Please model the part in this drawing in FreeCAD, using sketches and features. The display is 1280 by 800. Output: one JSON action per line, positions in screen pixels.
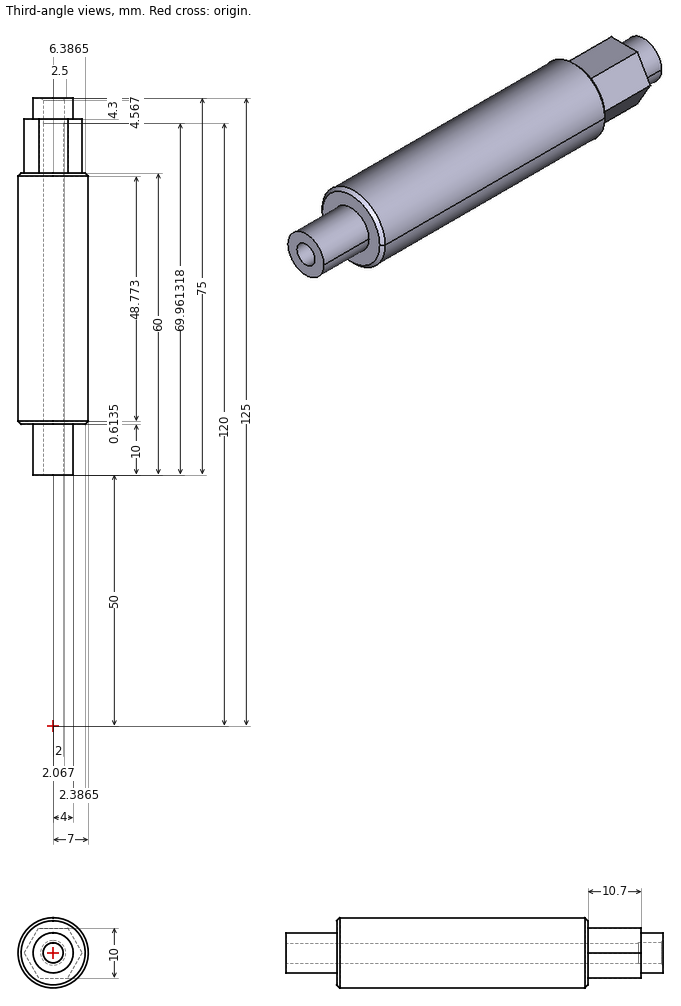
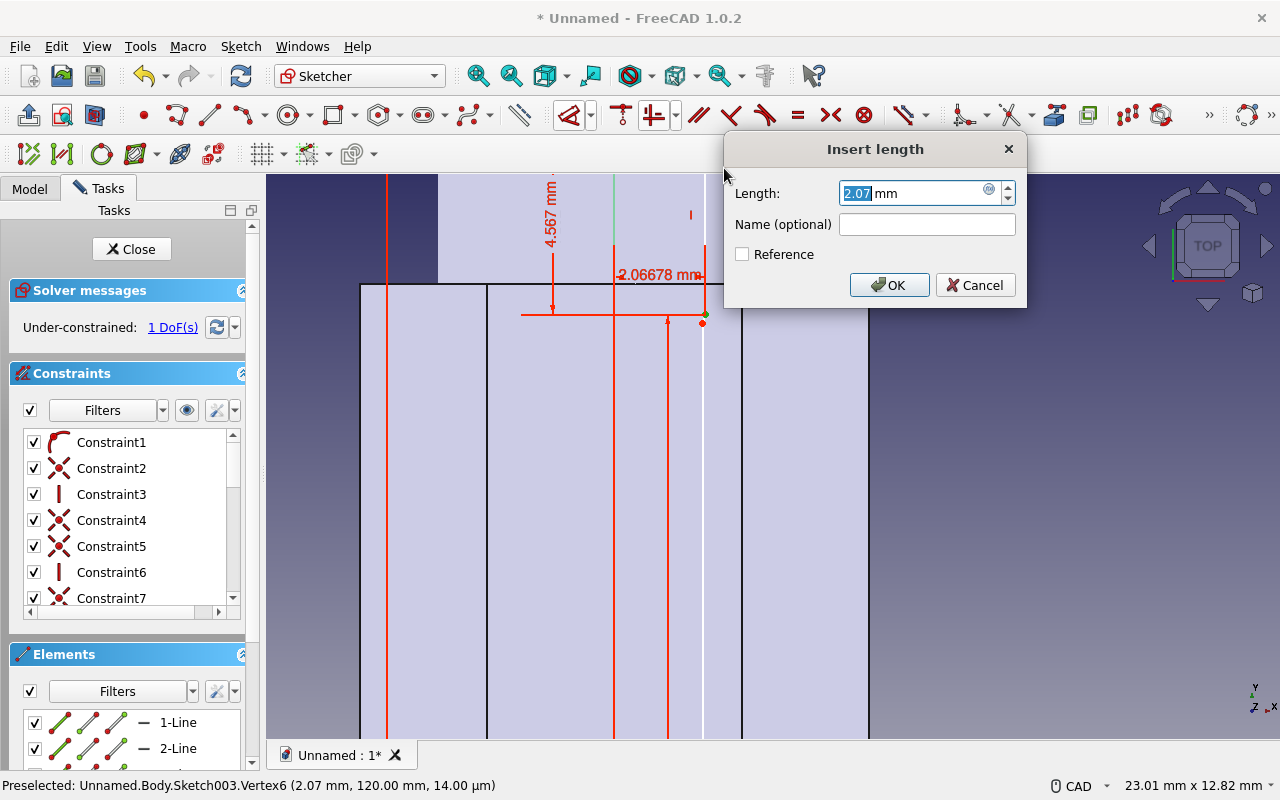
{"action": "type", "text": "2.067"}
{"action": "key", "text": "Return"}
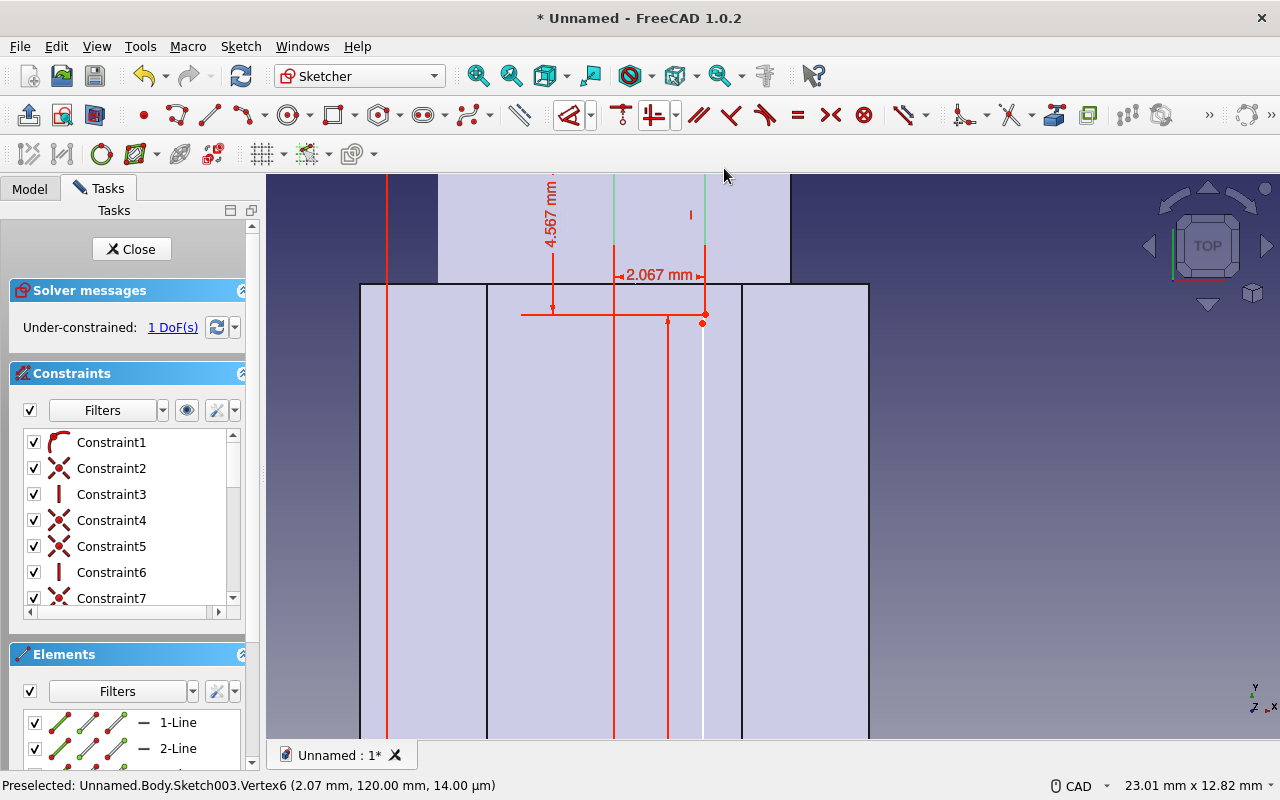
{"action": "scroll", "coordinate": [707, 302], "scroll_direction": "down", "scroll_amount": 14}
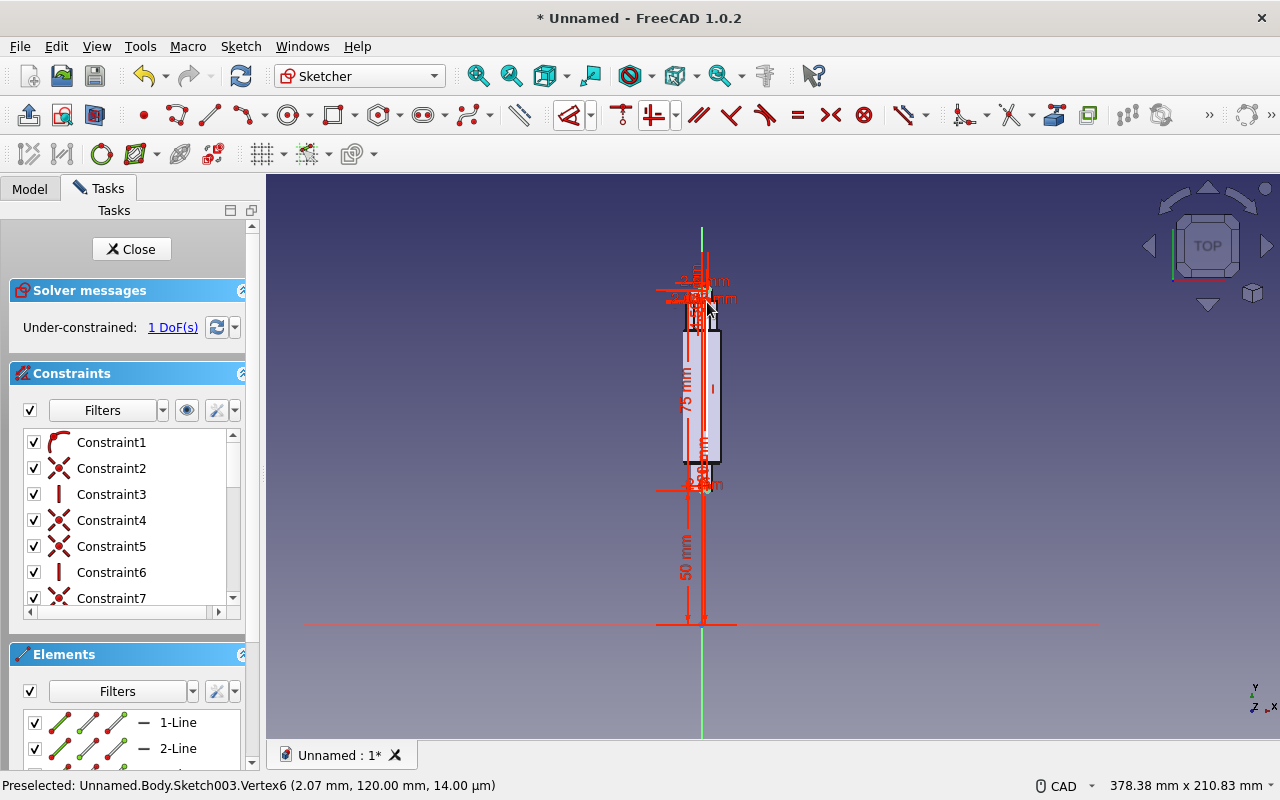
{"action": "scroll", "coordinate": [707, 434], "scroll_direction": "up", "scroll_amount": 5}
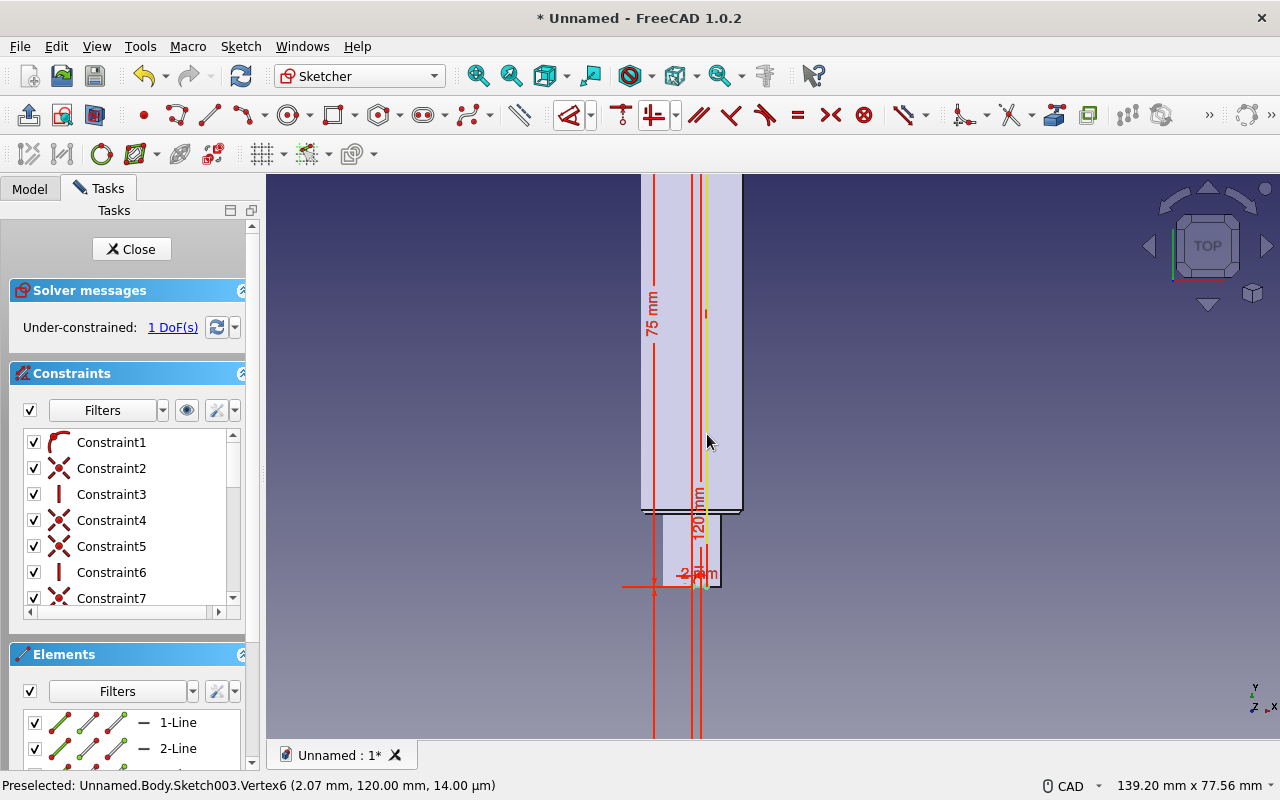
{"action": "left_click", "coordinate": [707, 434]}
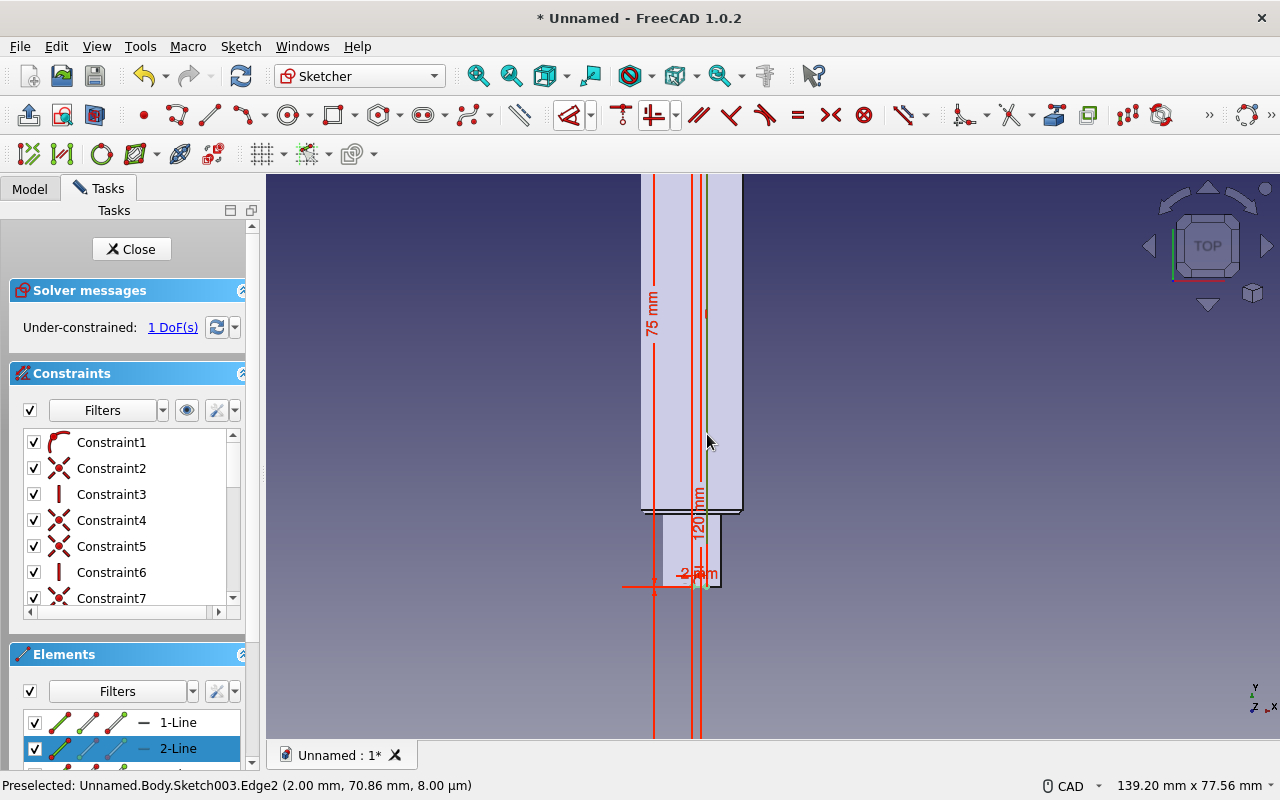
{"action": "key", "text": "i"}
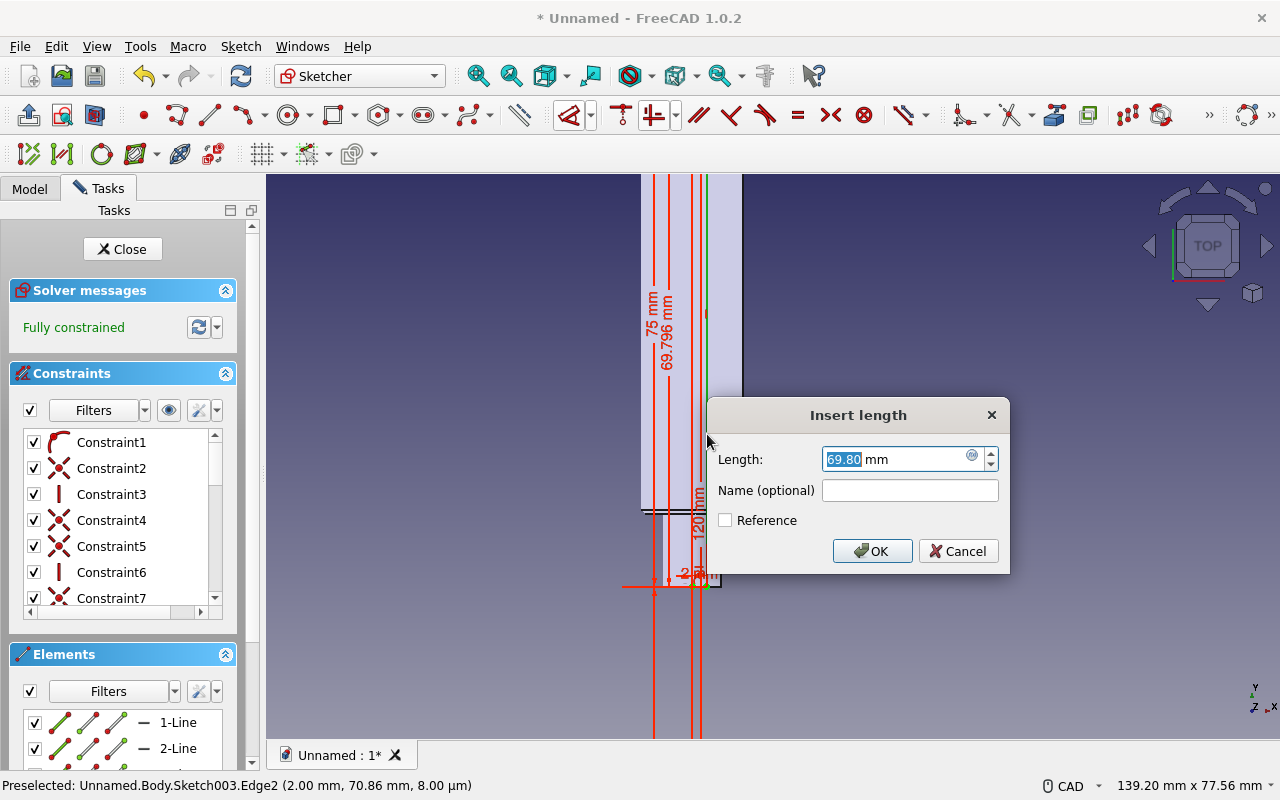
{"action": "type", "text": "69.961318"}
{"action": "key", "text": "Return"}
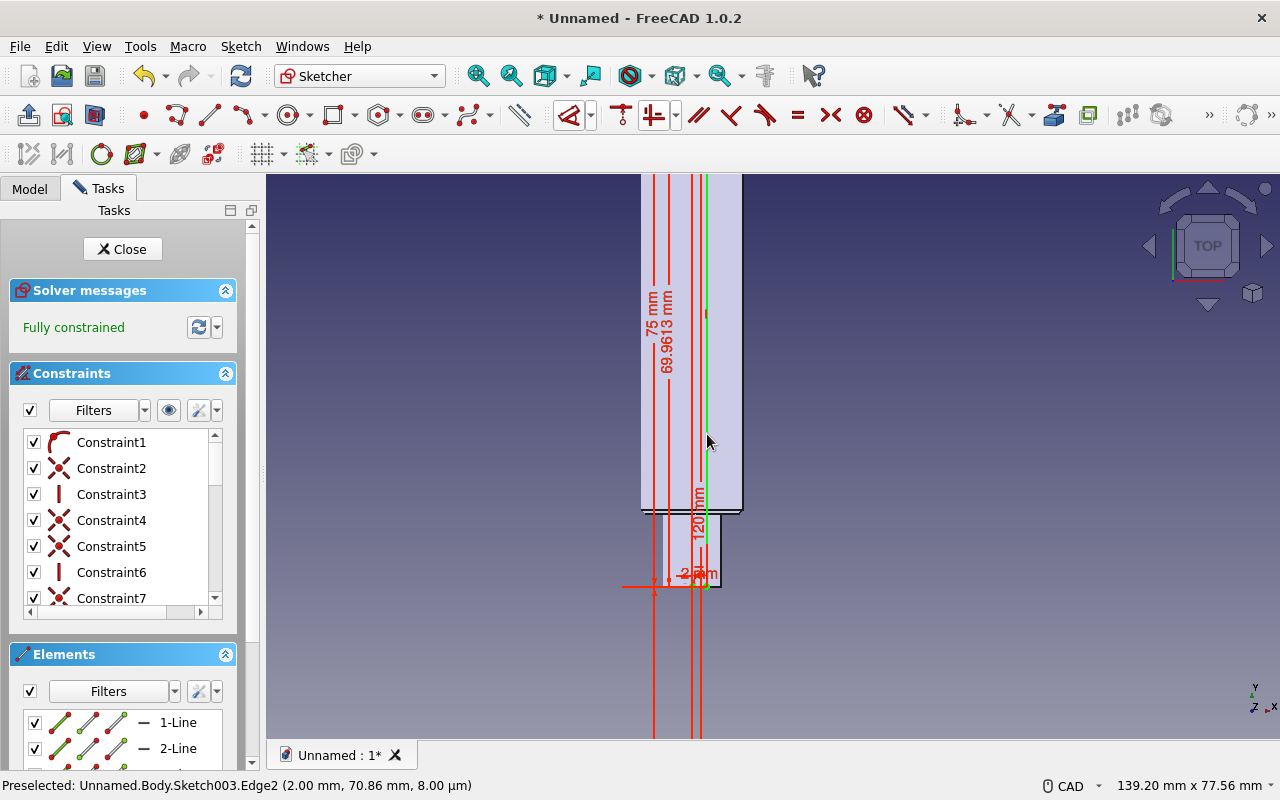
{"action": "left_click", "coordinate": [123, 249]}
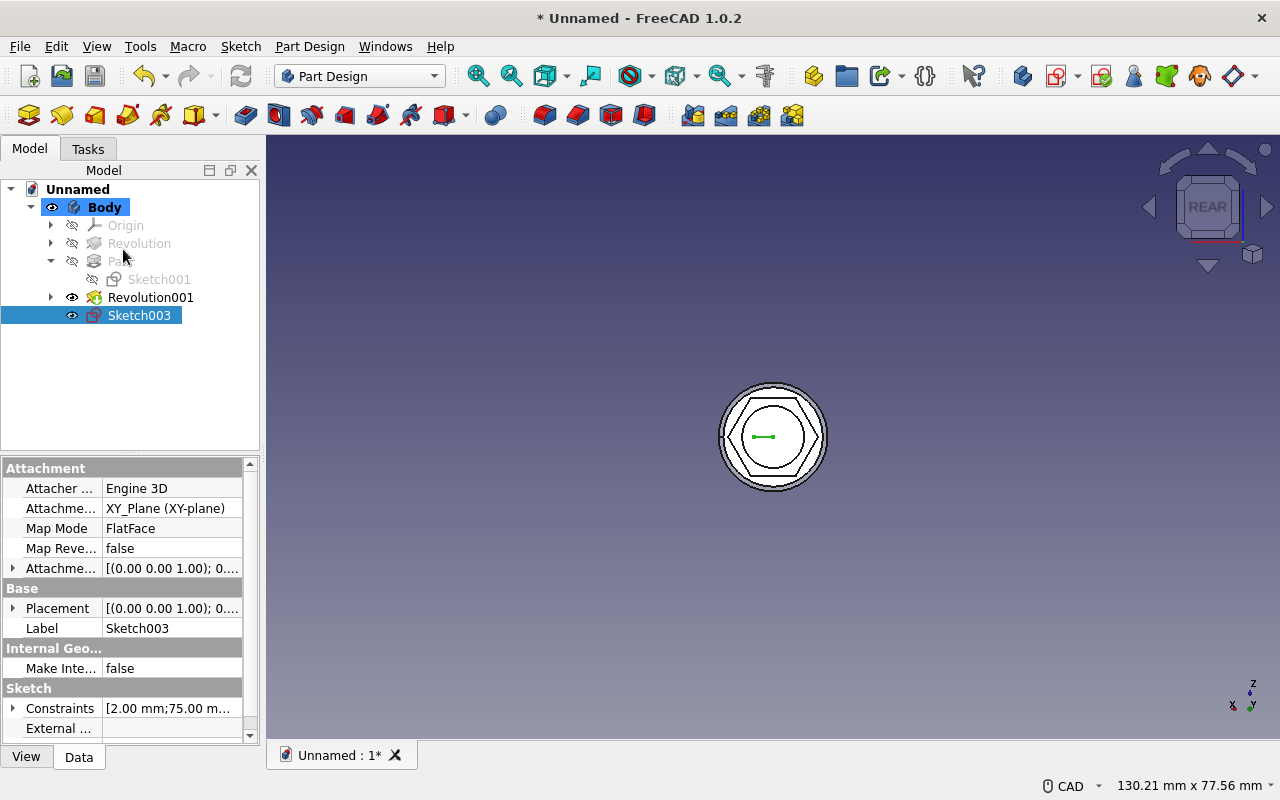
{"action": "left_click", "coordinate": [312, 116]}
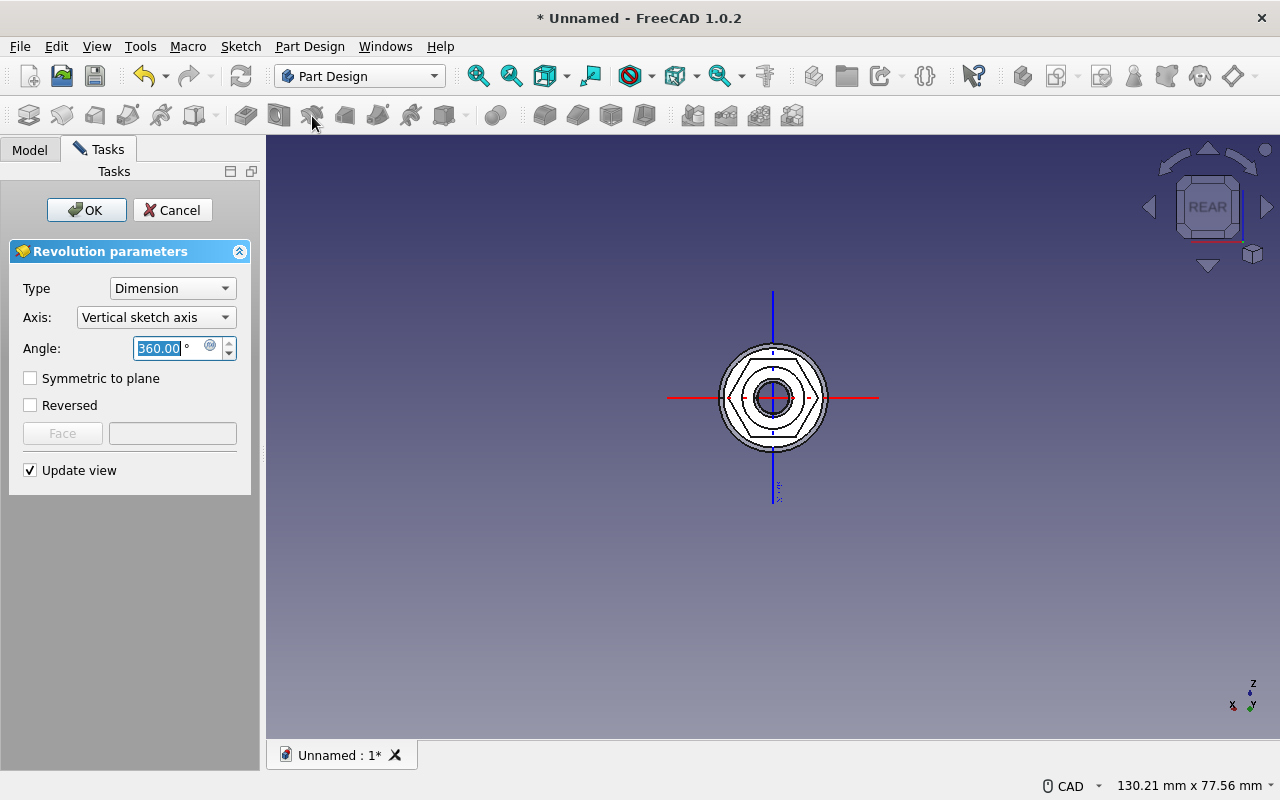
{"action": "left_click", "coordinate": [87, 210]}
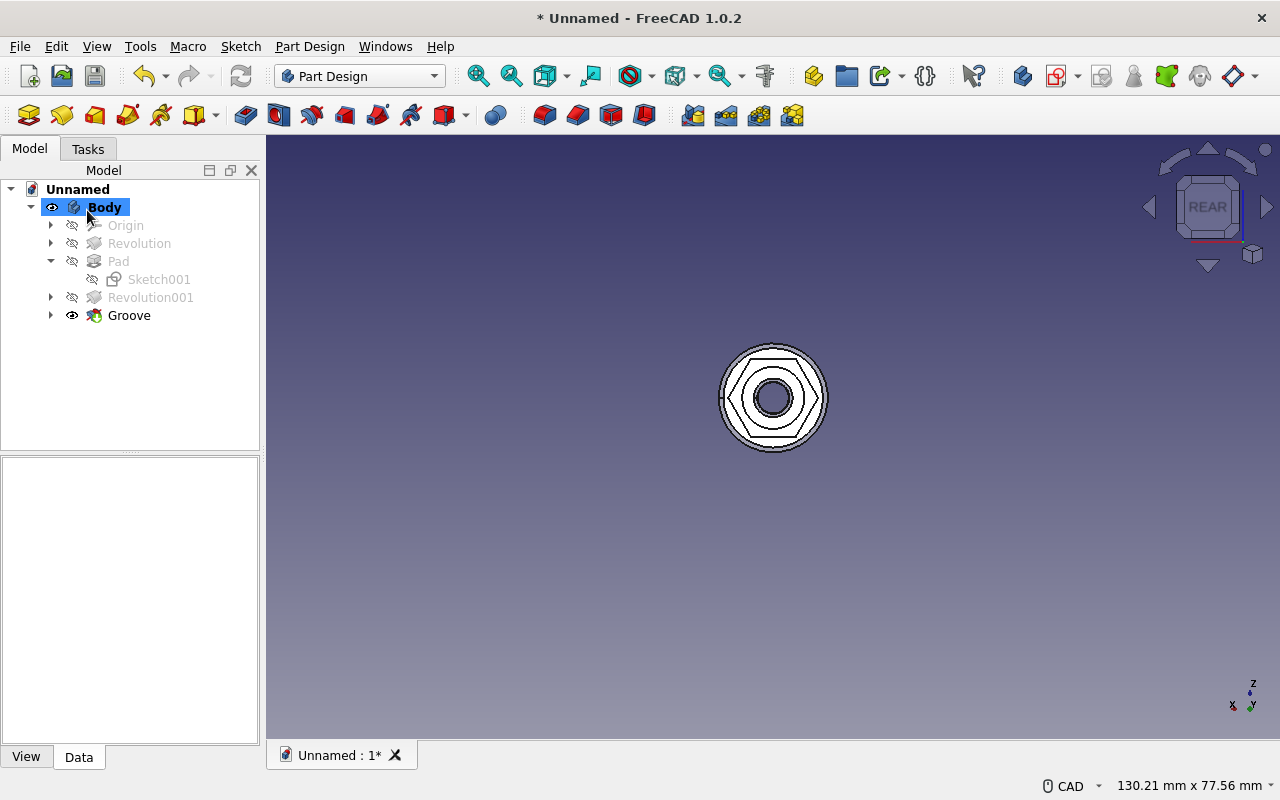
{"action": "key", "text": "0"}